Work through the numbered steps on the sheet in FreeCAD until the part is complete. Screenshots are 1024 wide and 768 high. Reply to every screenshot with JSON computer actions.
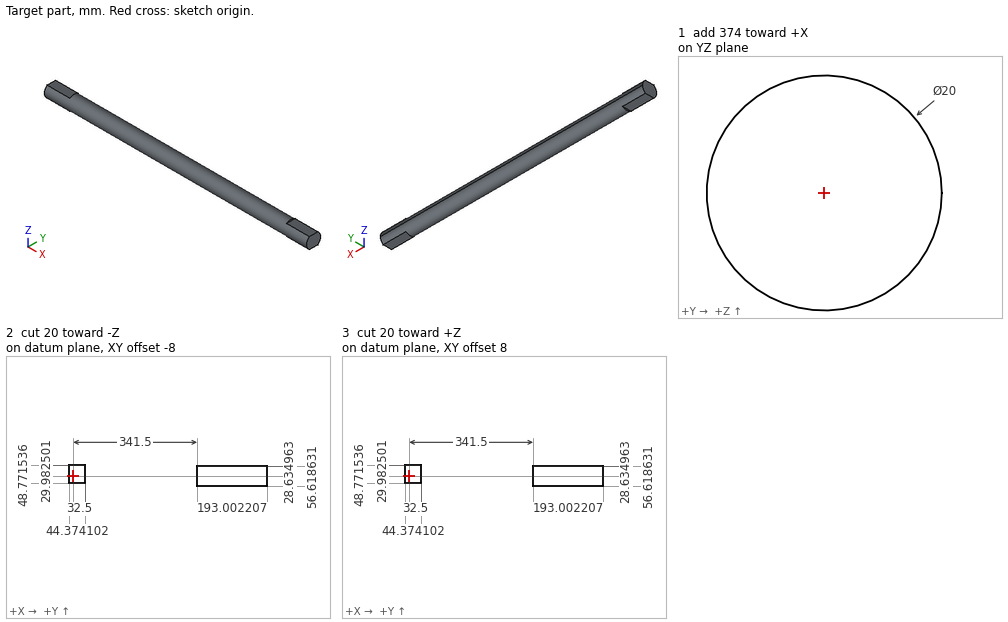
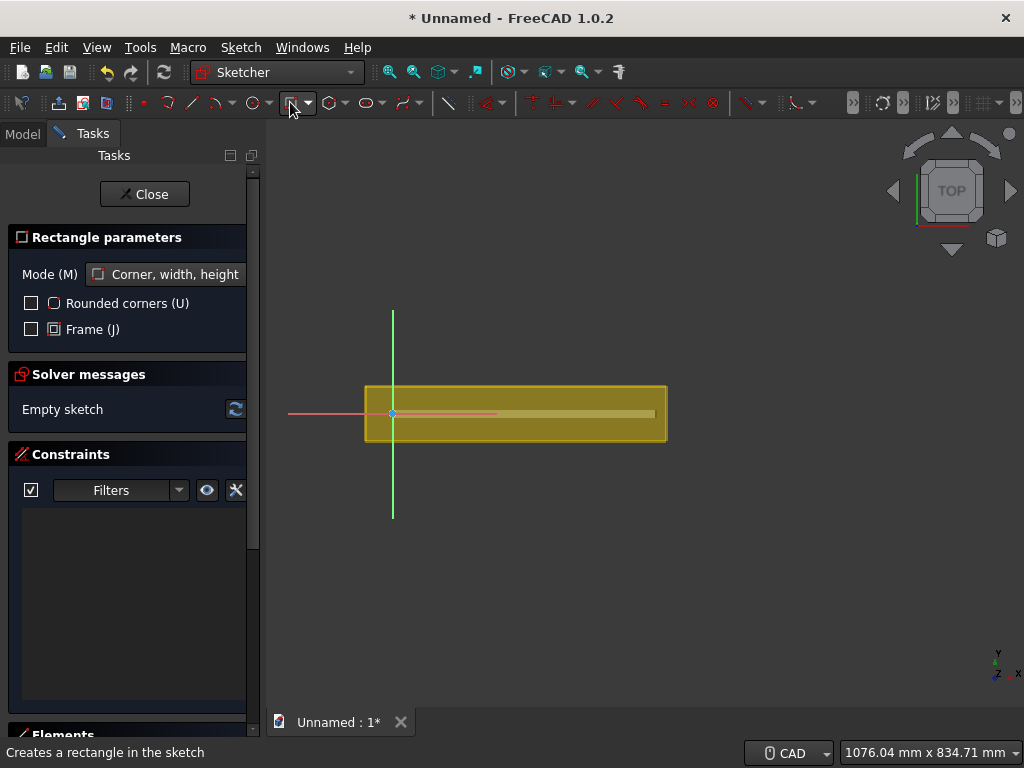
{"action": "scroll", "coordinate": [384, 393], "scroll_direction": "up", "scroll_amount": 4}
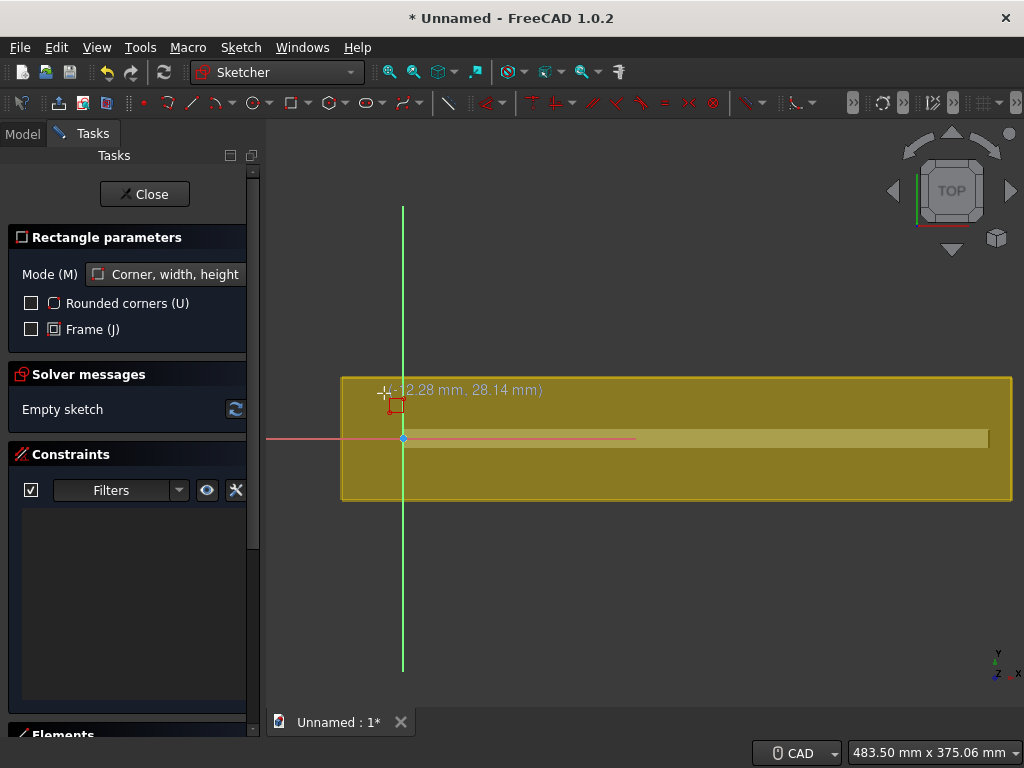
{"action": "left_click", "coordinate": [384, 392]}
{"action": "mouse_move", "coordinate": [454, 468]}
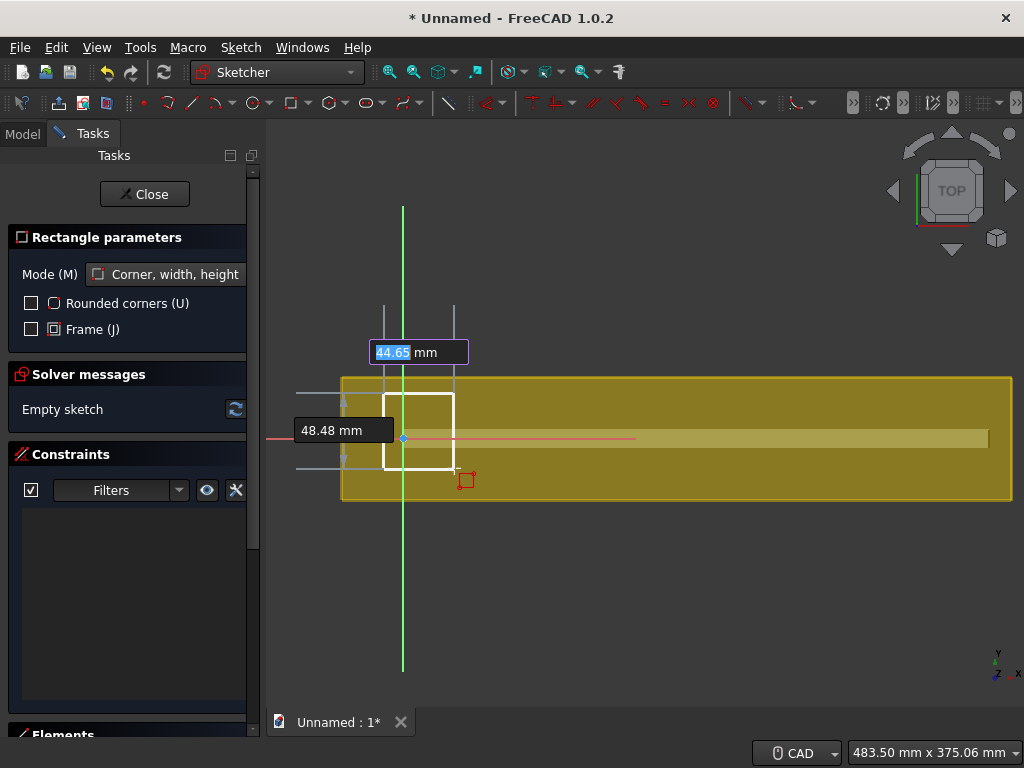
{"action": "type", "text": "44.374102"}
{"action": "key", "text": "Tab"}
{"action": "type", "text": "48.771536"}
{"action": "key", "text": "Return"}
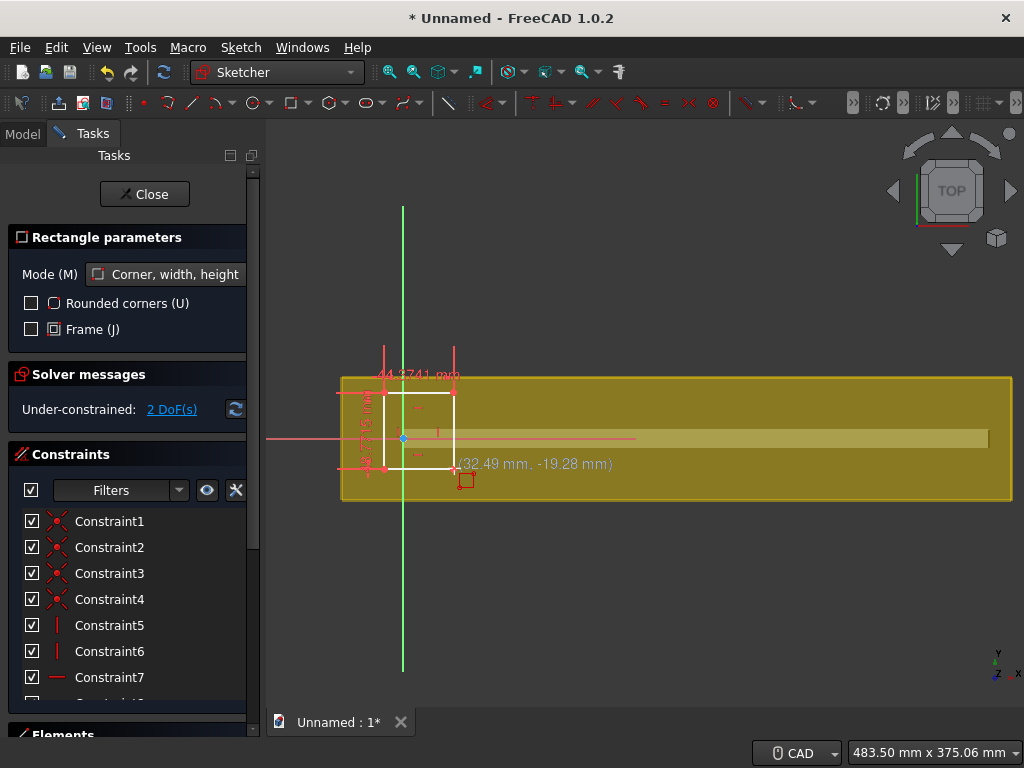
{"action": "scroll", "coordinate": [384, 393], "scroll_direction": "down", "scroll_amount": 4}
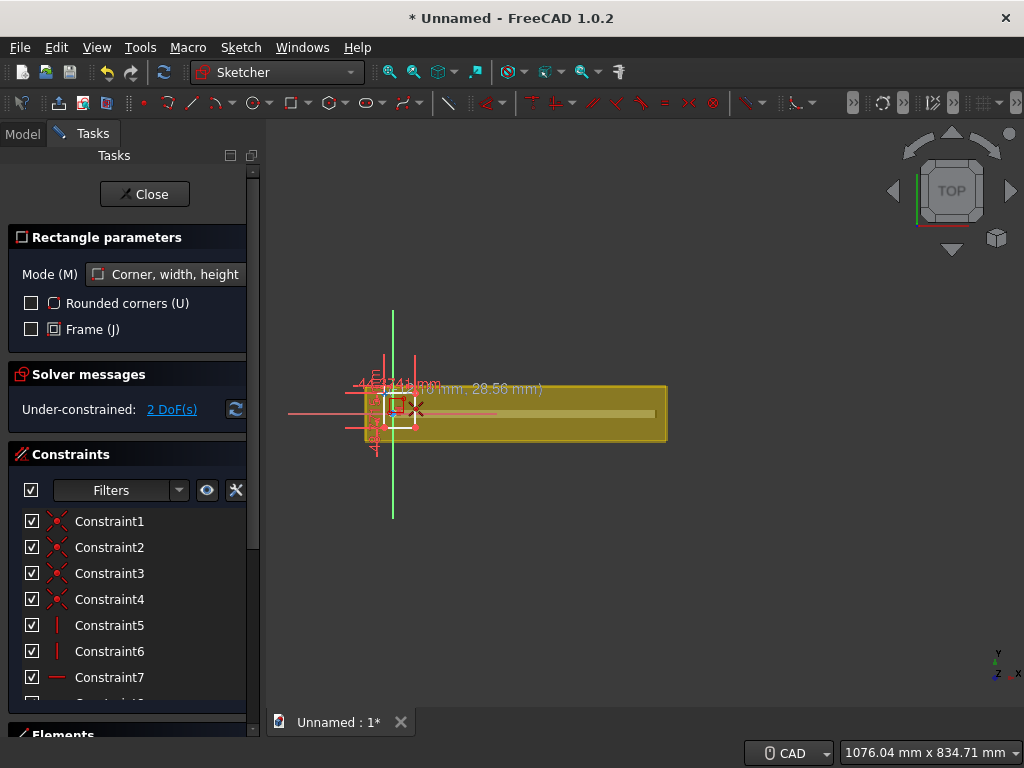
{"action": "left_click", "coordinate": [633, 394]}
{"action": "mouse_move", "coordinate": [769, 434]}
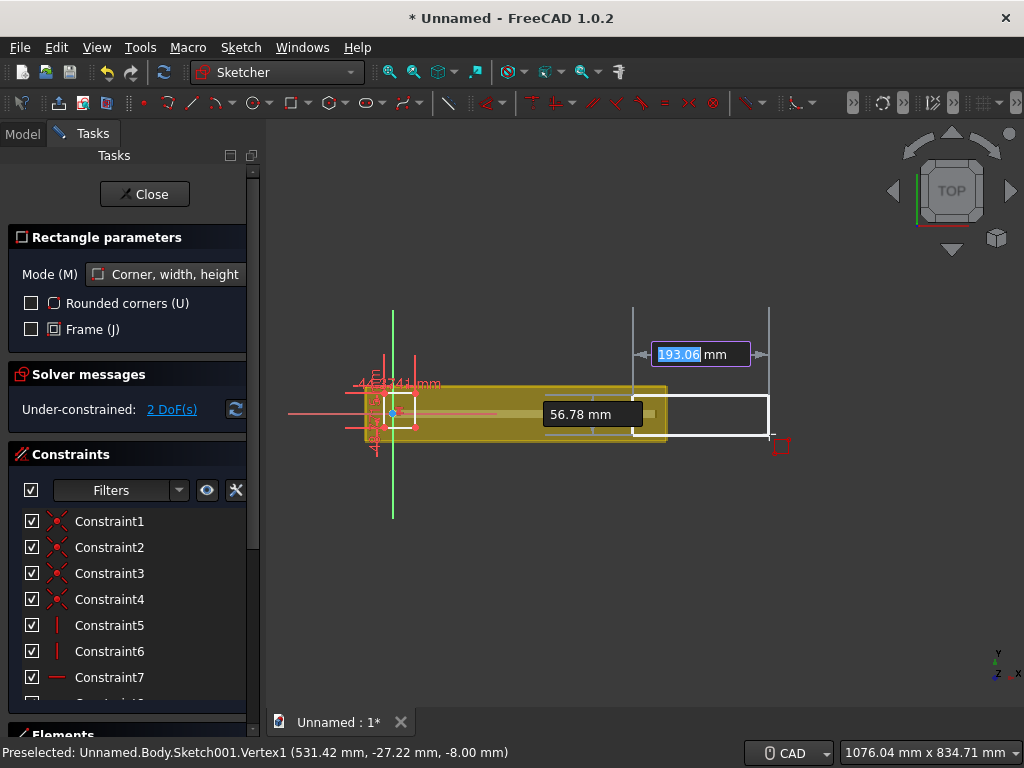
{"action": "type", "text": "193.002207"}
{"action": "key", "text": "Tab"}
{"action": "type", "text": "56.618631"}
{"action": "key", "text": "Return"}
{"action": "key", "text": "Escape"}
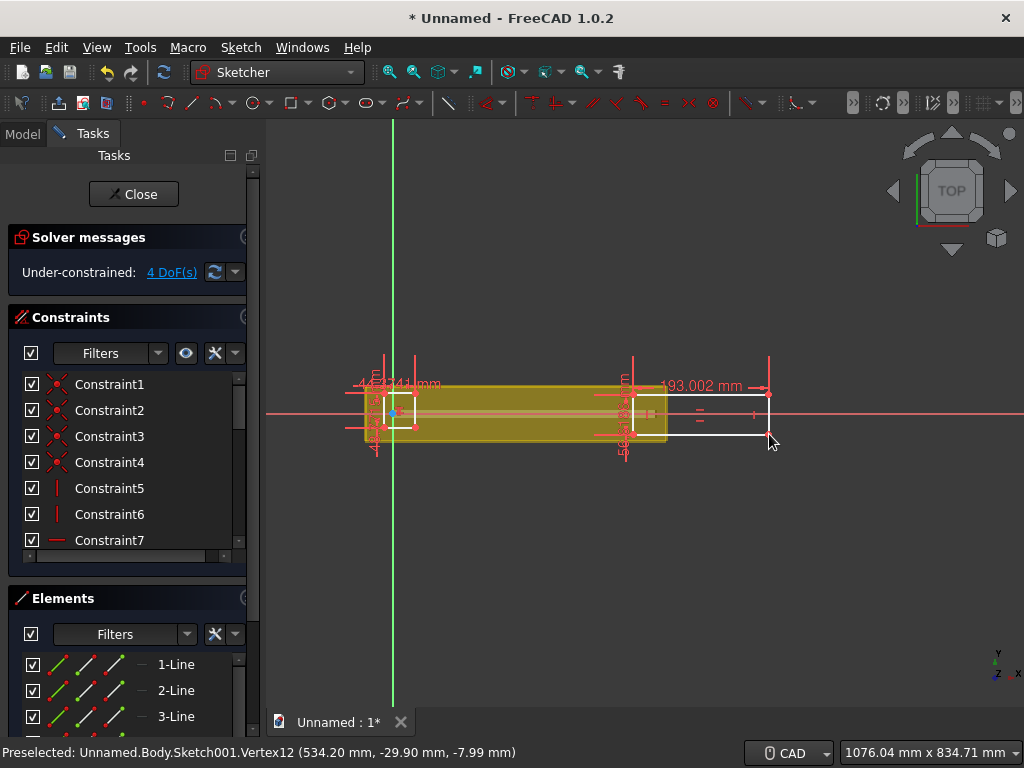
{"action": "scroll", "coordinate": [415, 428], "scroll_direction": "up", "scroll_amount": 3}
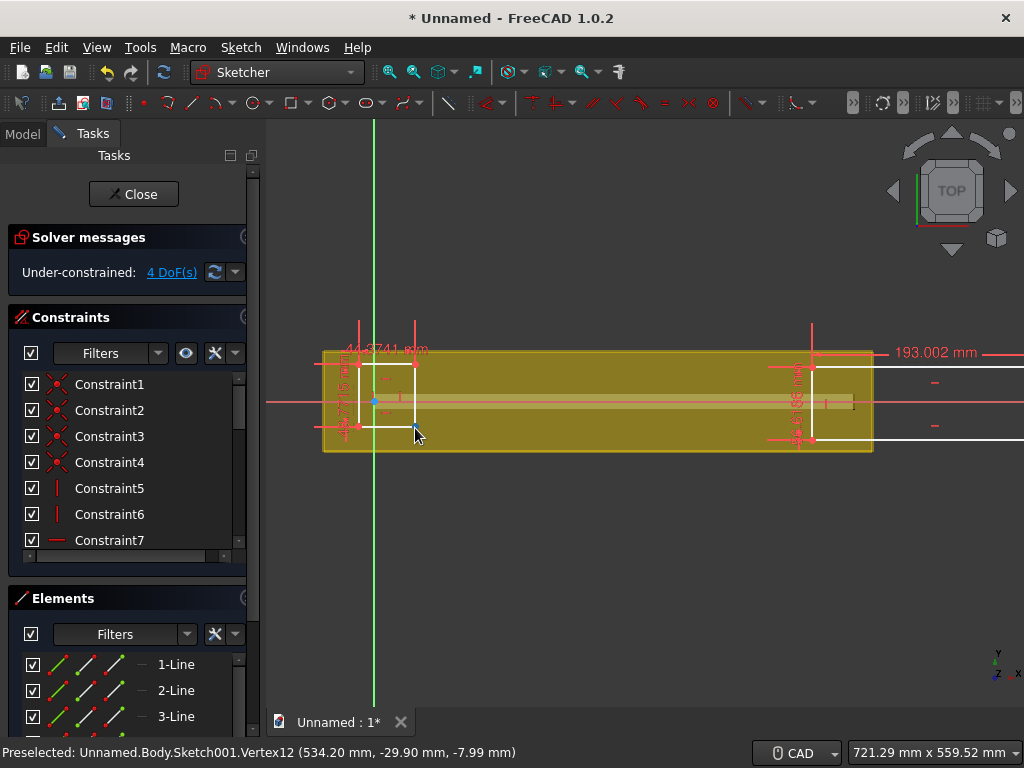
{"action": "left_click", "coordinate": [415, 427]}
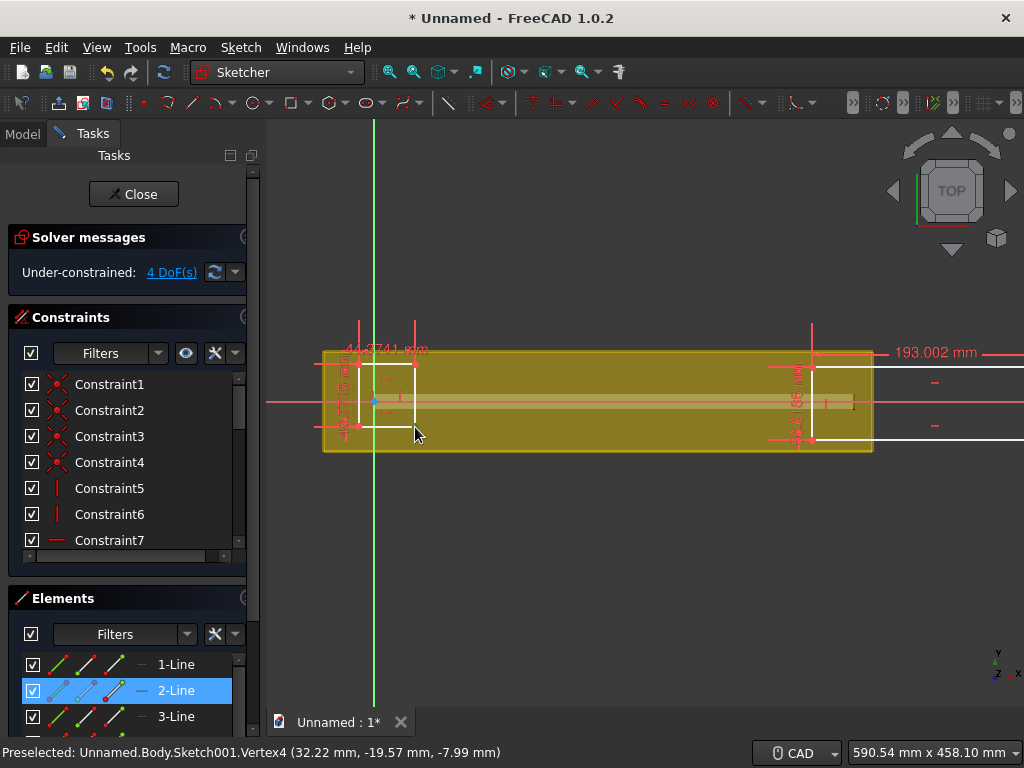
{"action": "left_click", "coordinate": [504, 104]}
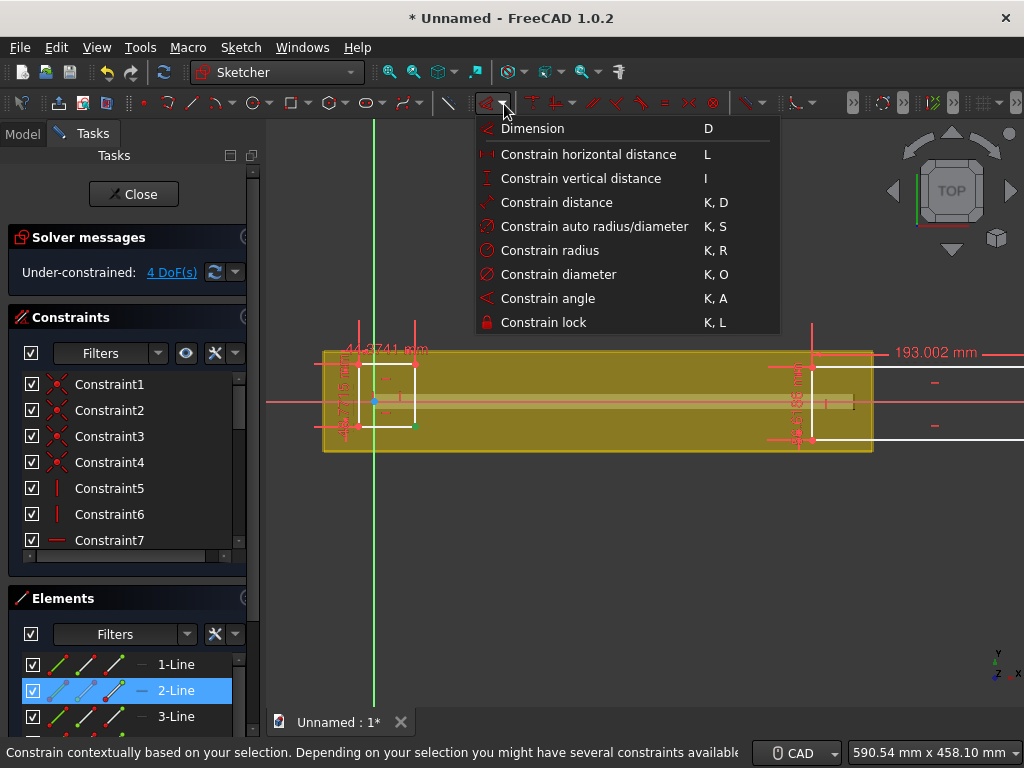
{"action": "left_click", "coordinate": [628, 154]}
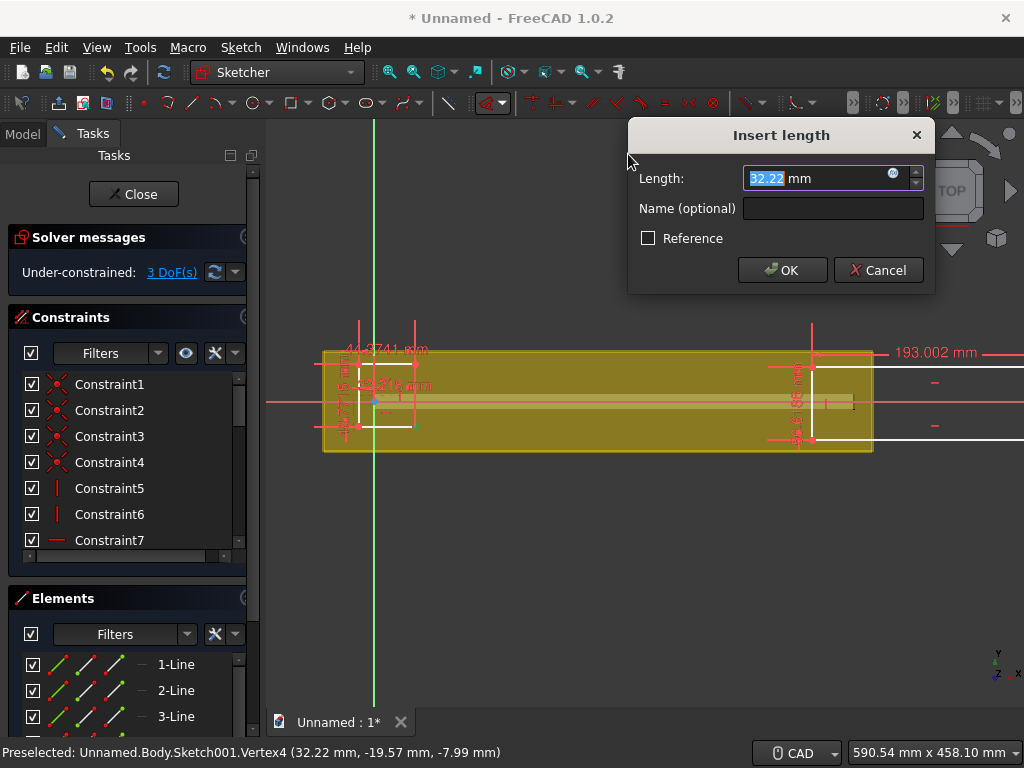
{"action": "type", "text": "32.5"}
{"action": "key", "text": "Return"}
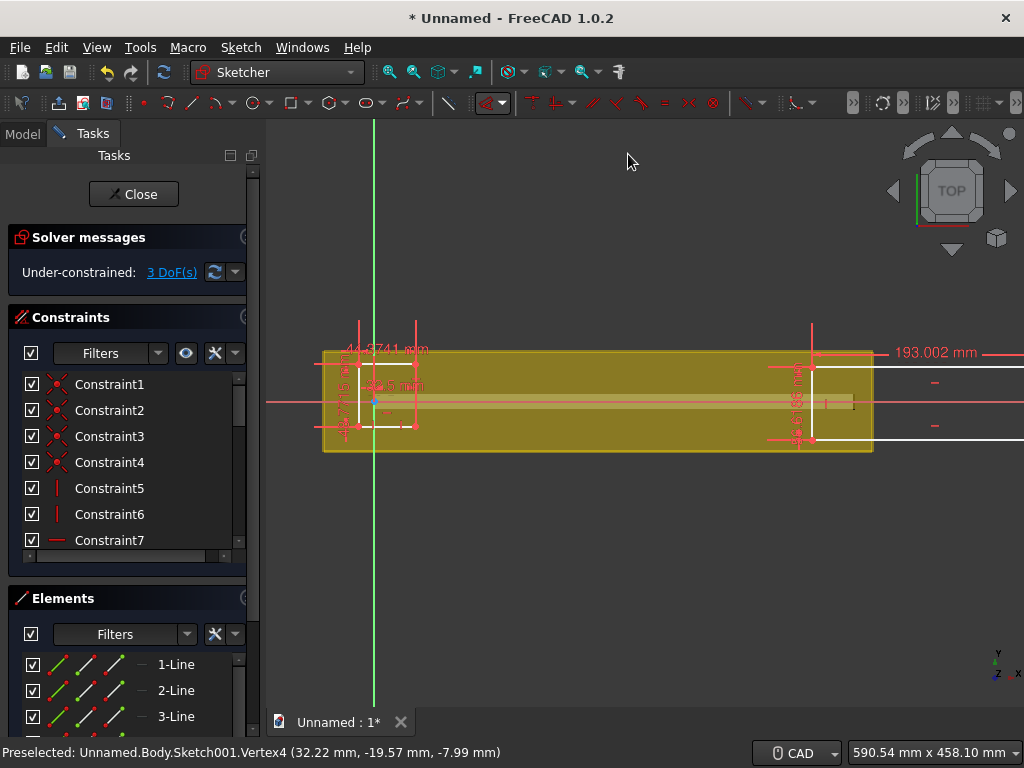
{"action": "left_click", "coordinate": [812, 367]}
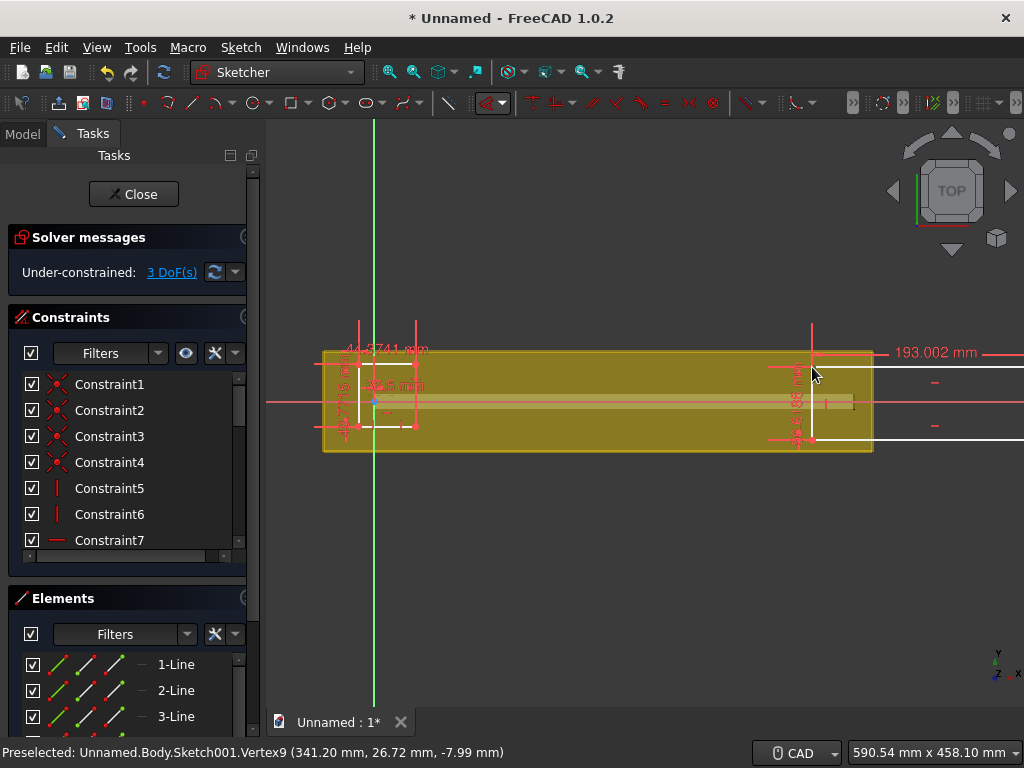
{"action": "left_click", "coordinate": [504, 104]}